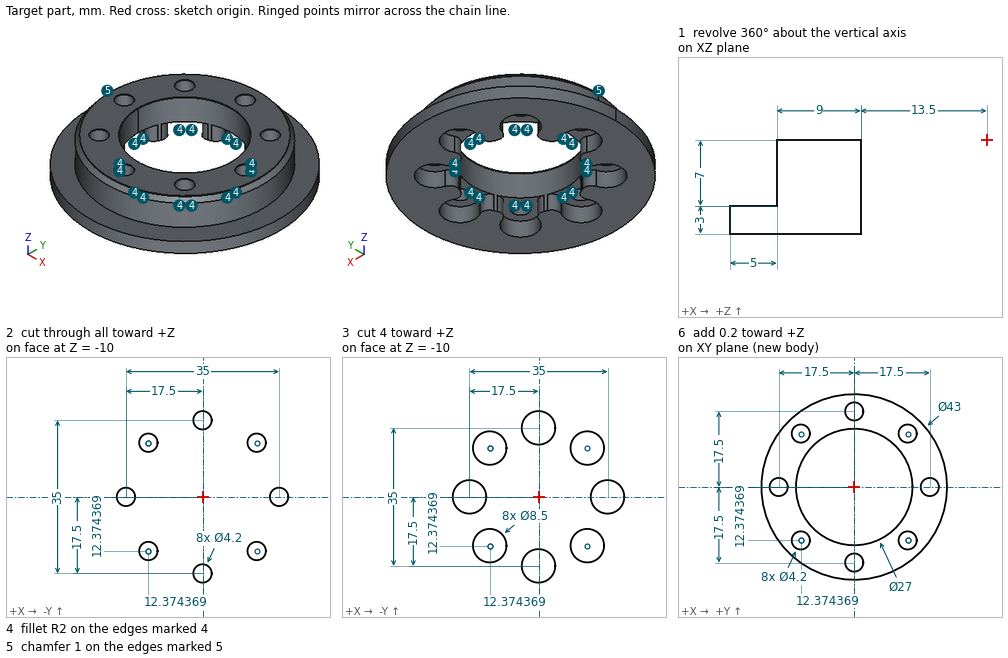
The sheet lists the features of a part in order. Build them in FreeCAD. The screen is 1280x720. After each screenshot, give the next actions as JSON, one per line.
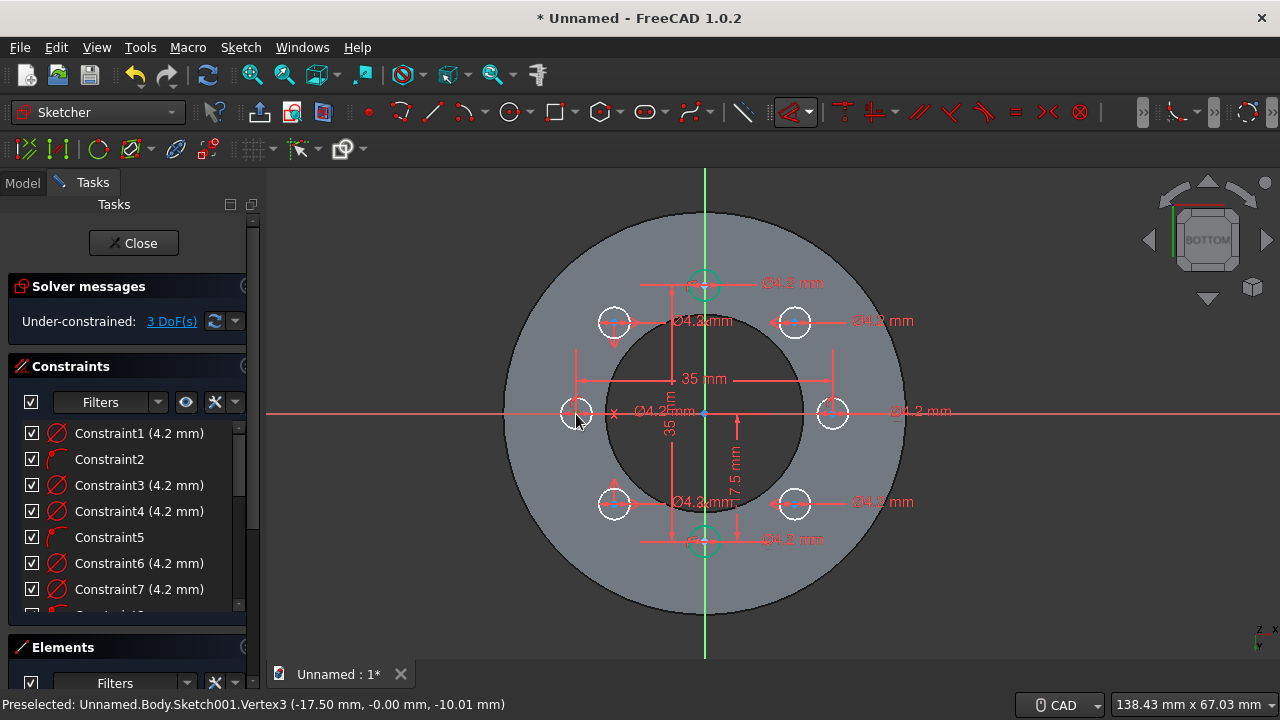
{"action": "left_click", "coordinate": [812, 112]}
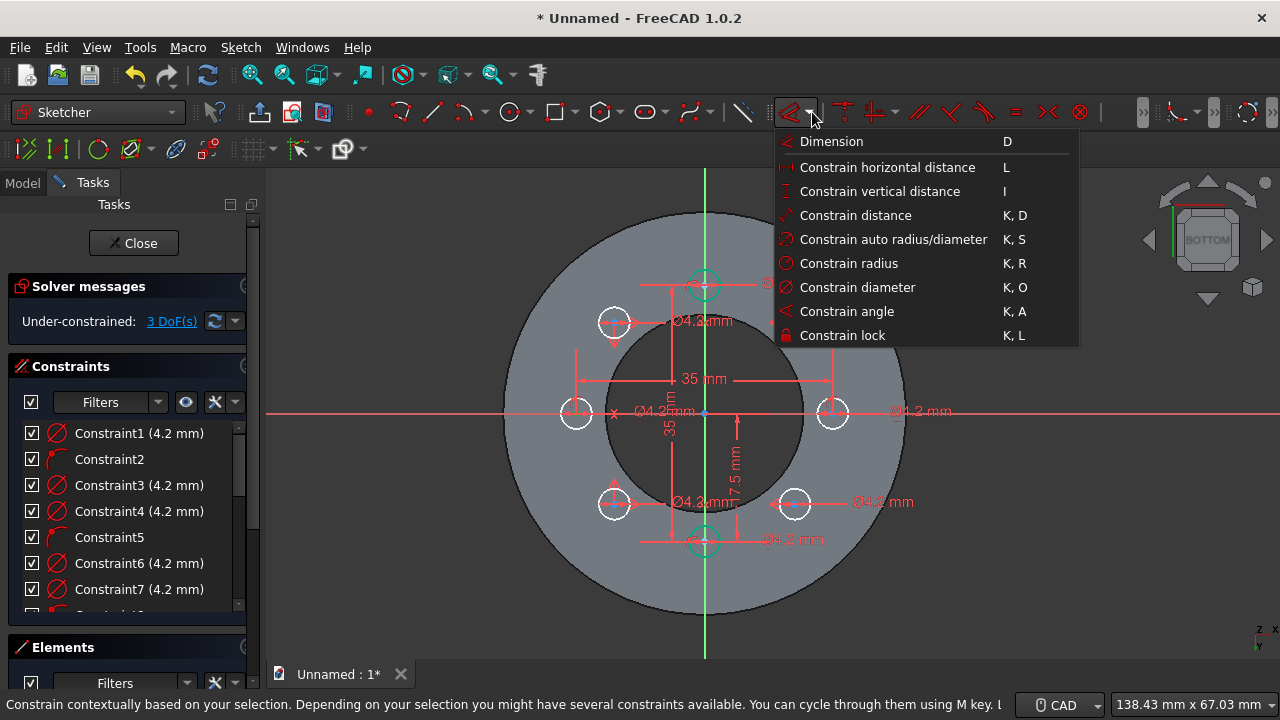
{"action": "left_click", "coordinate": [927, 167]}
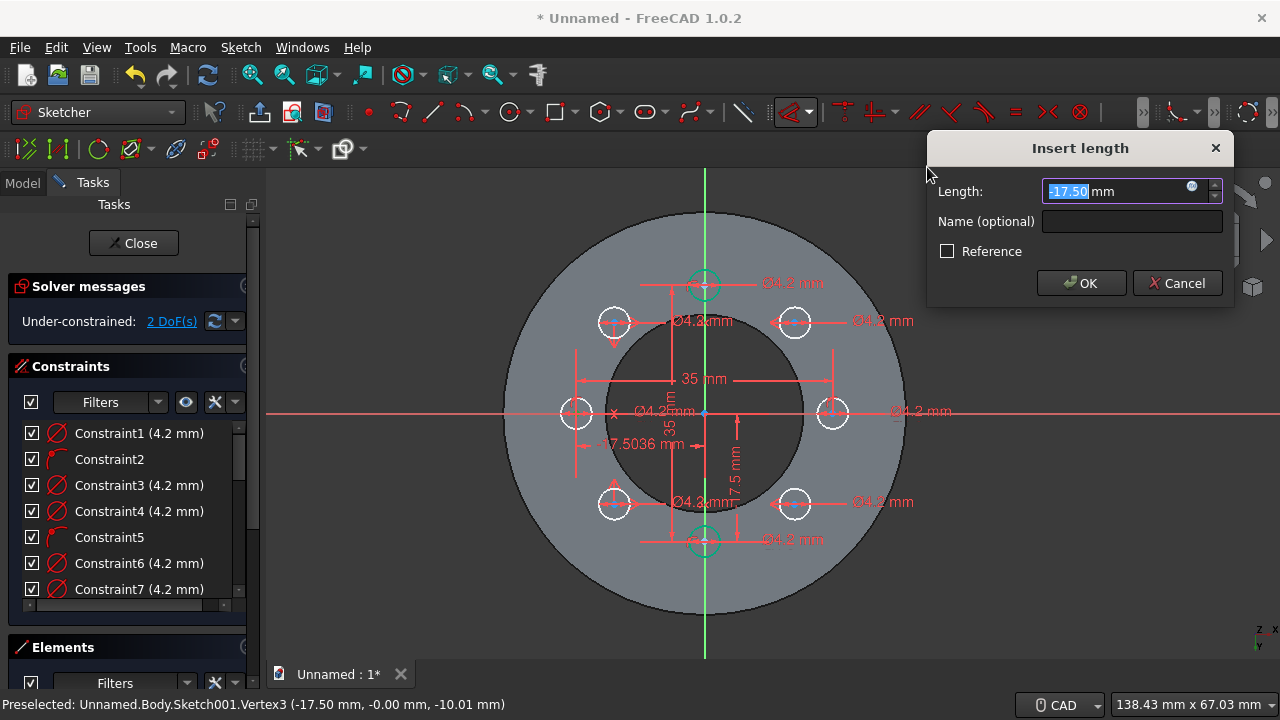
{"action": "type", "text": "-17.5"}
{"action": "key", "text": "Return"}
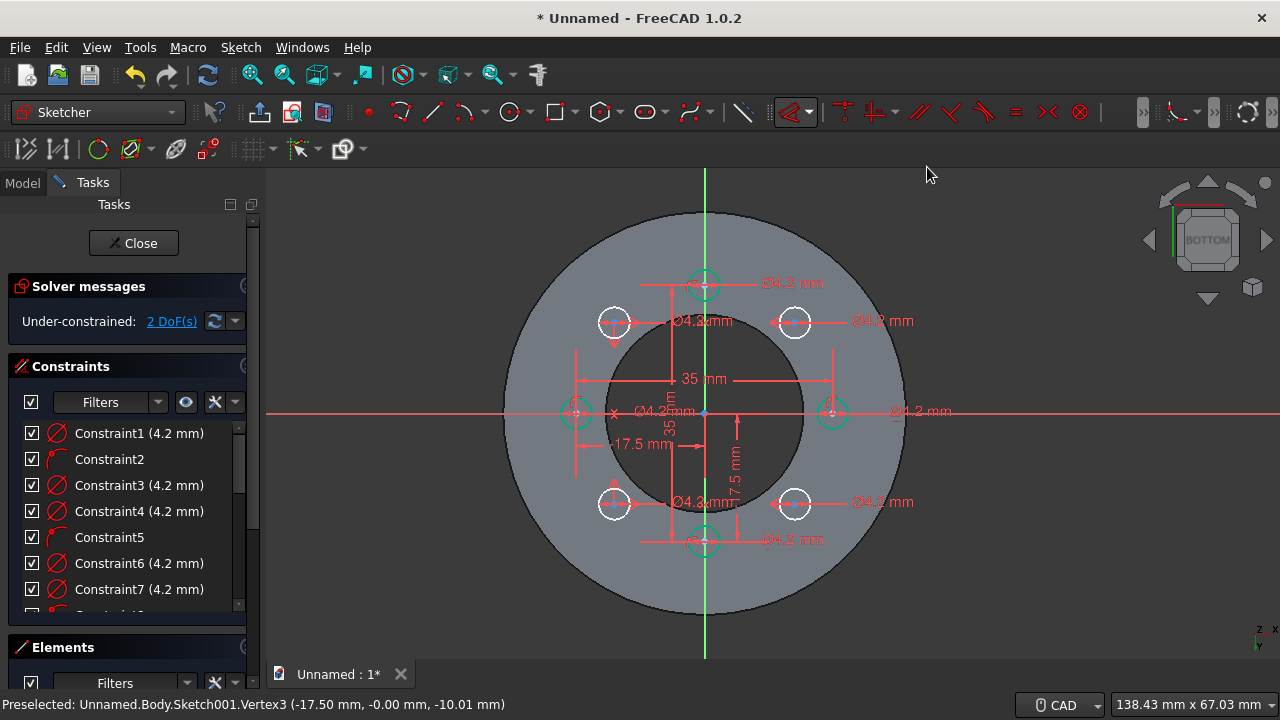
{"action": "left_click", "coordinate": [614, 504]}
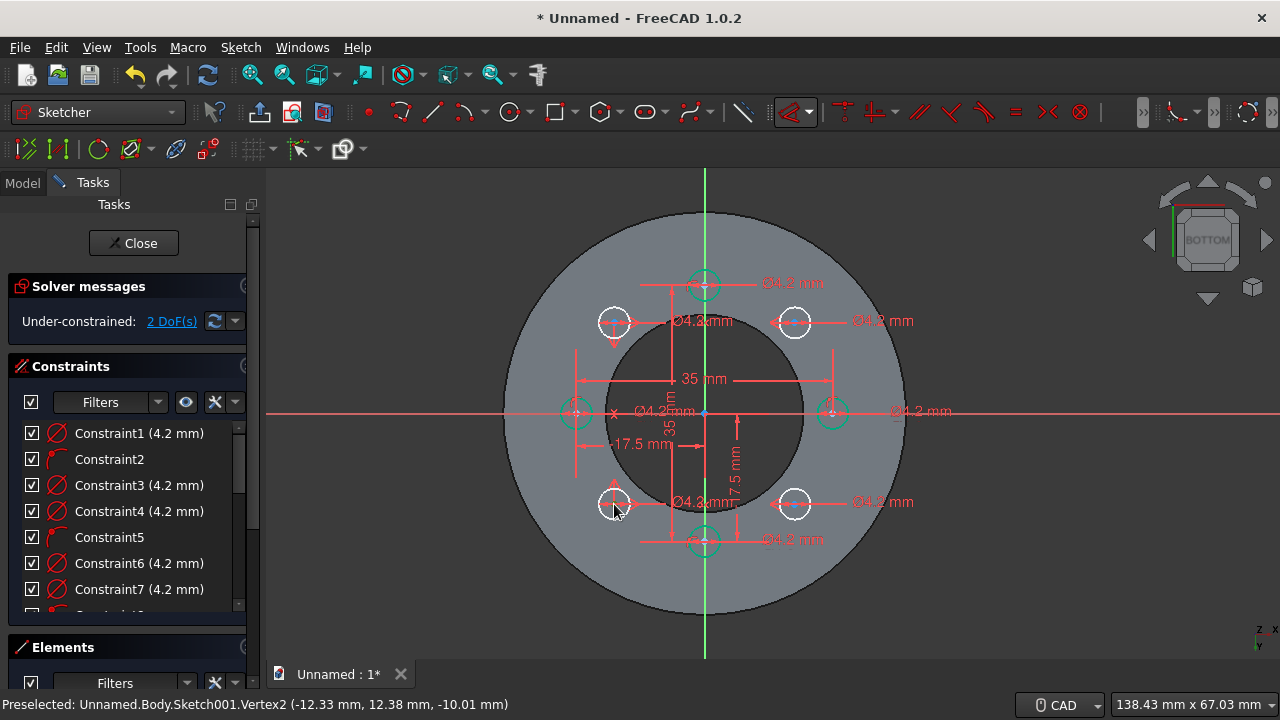
{"action": "key", "text": "l"}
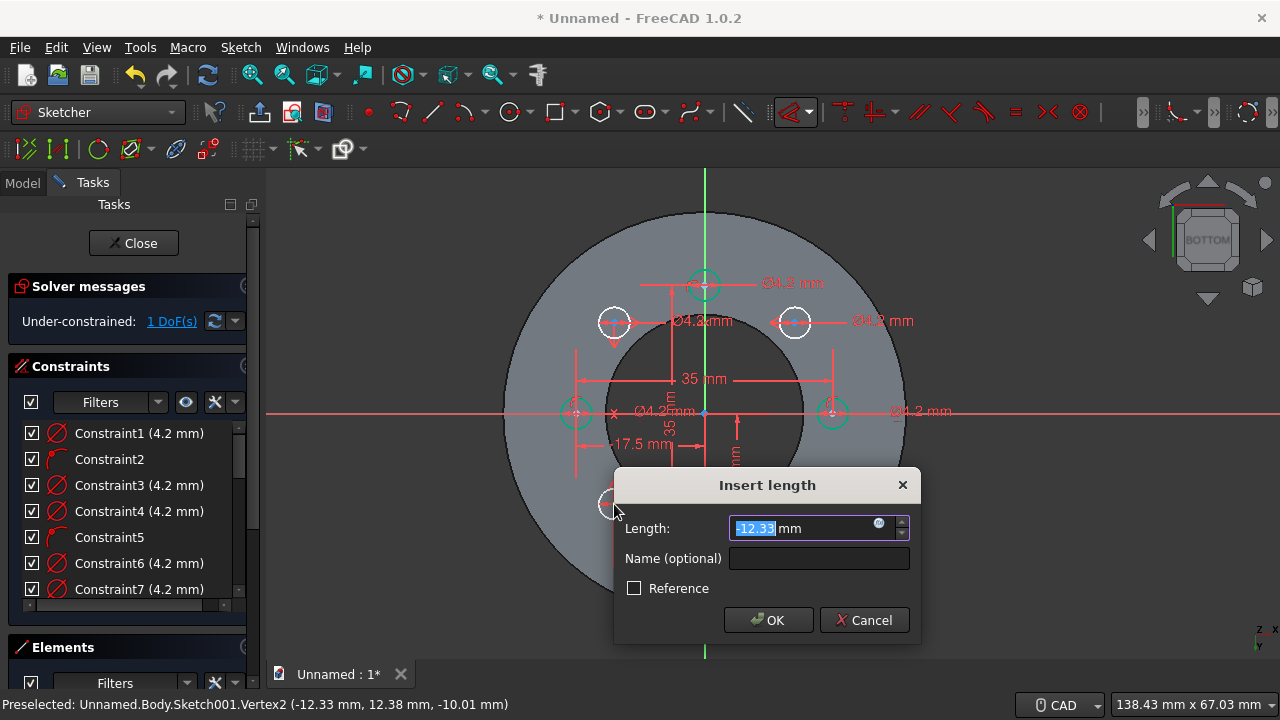
{"action": "type", "text": "-12.374369"}
{"action": "key", "text": "Return"}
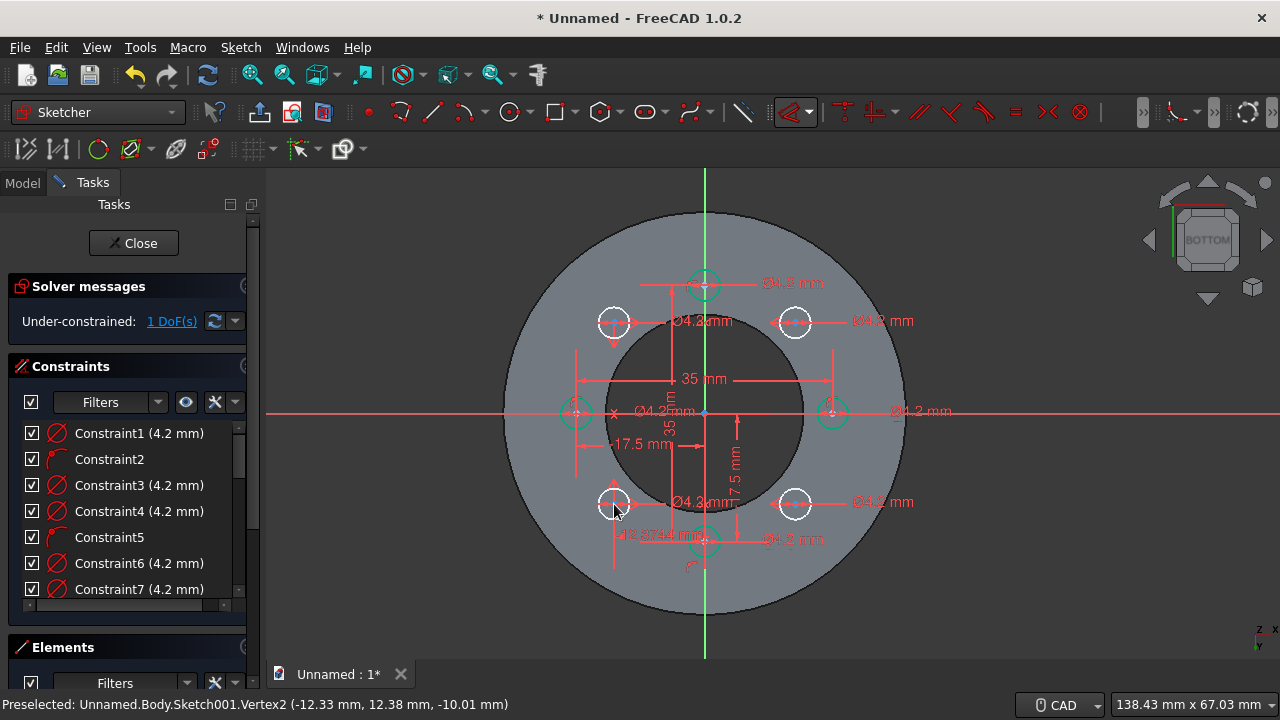
{"action": "left_click", "coordinate": [614, 504]}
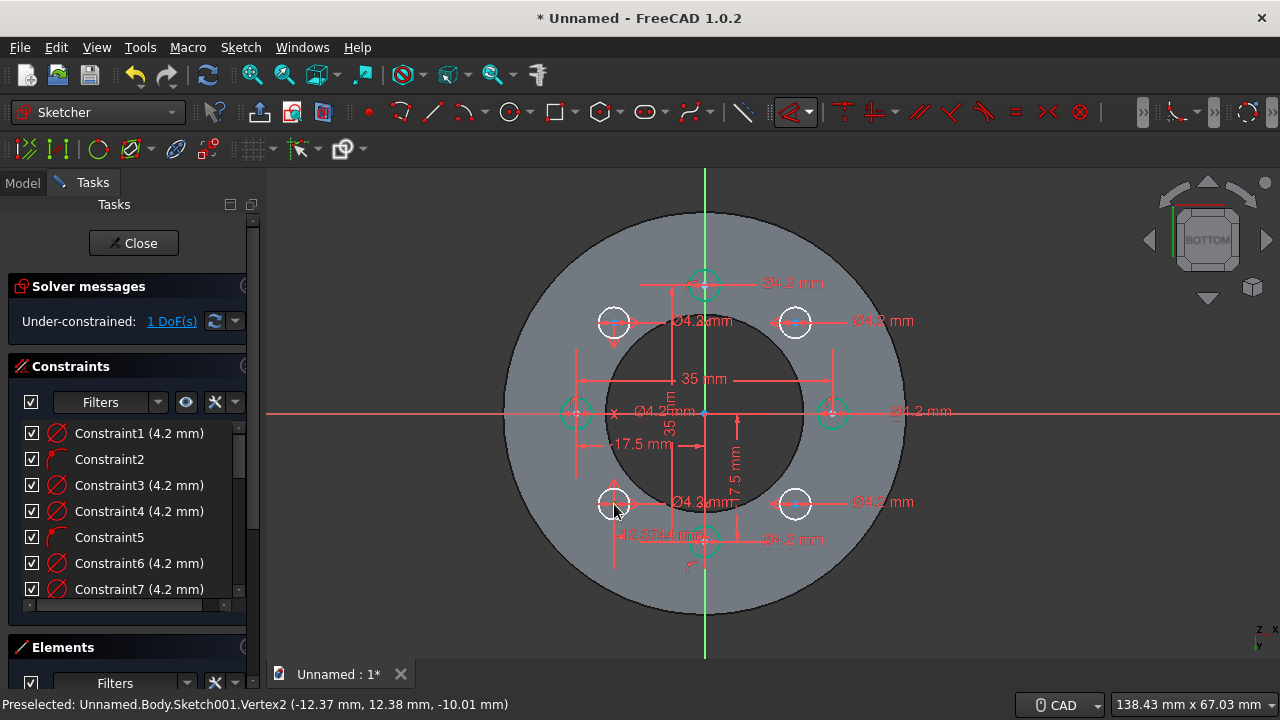
{"action": "key", "text": "i"}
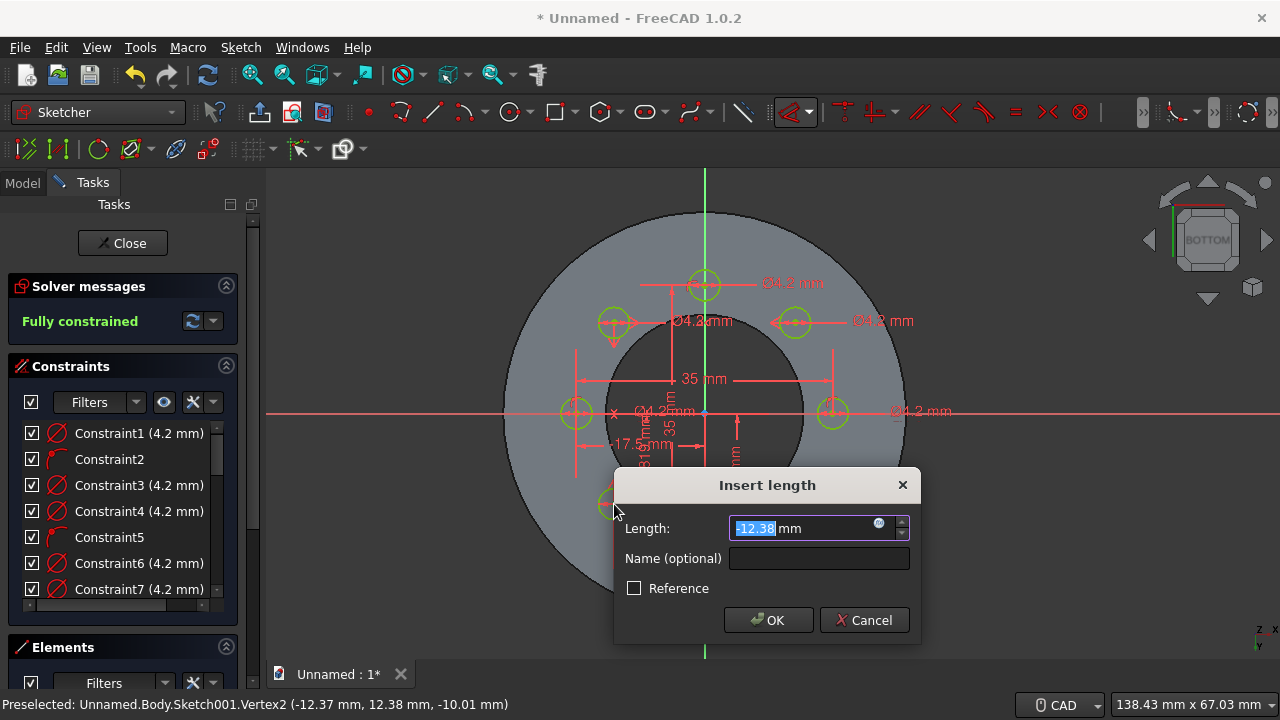
{"action": "type", "text": "-12.374369"}
{"action": "key", "text": "Return"}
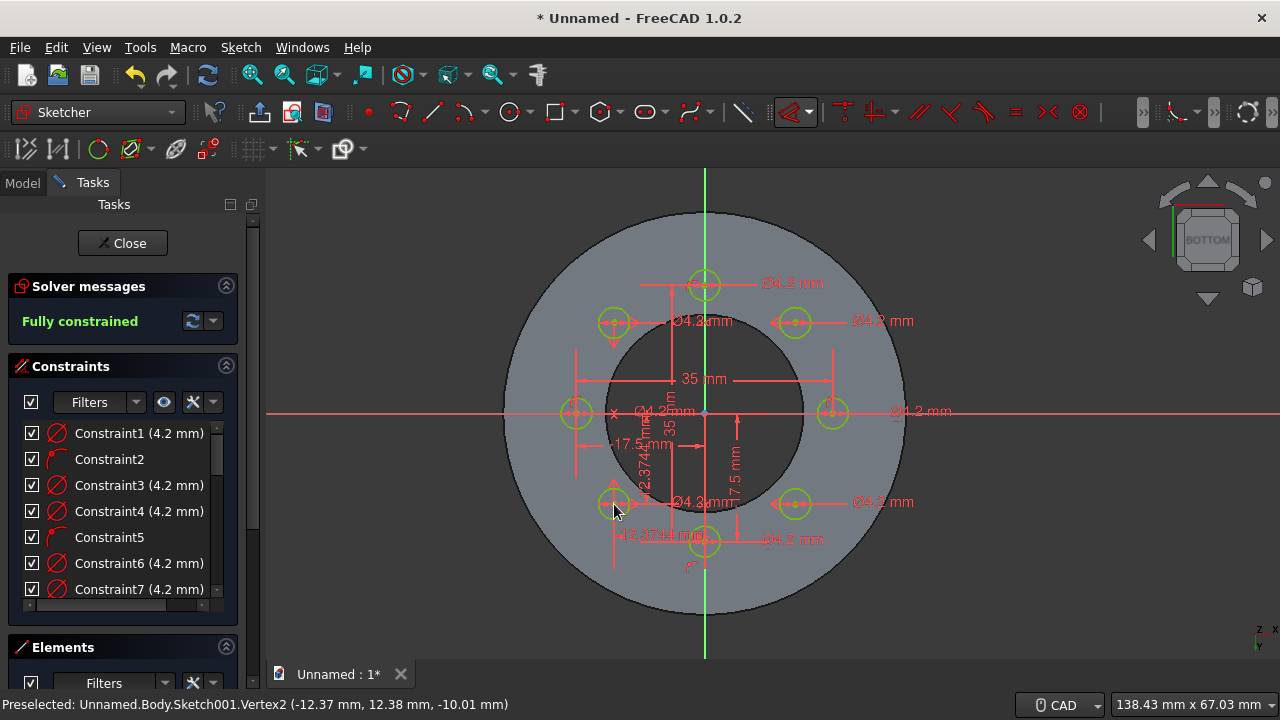
{"action": "left_click", "coordinate": [123, 243]}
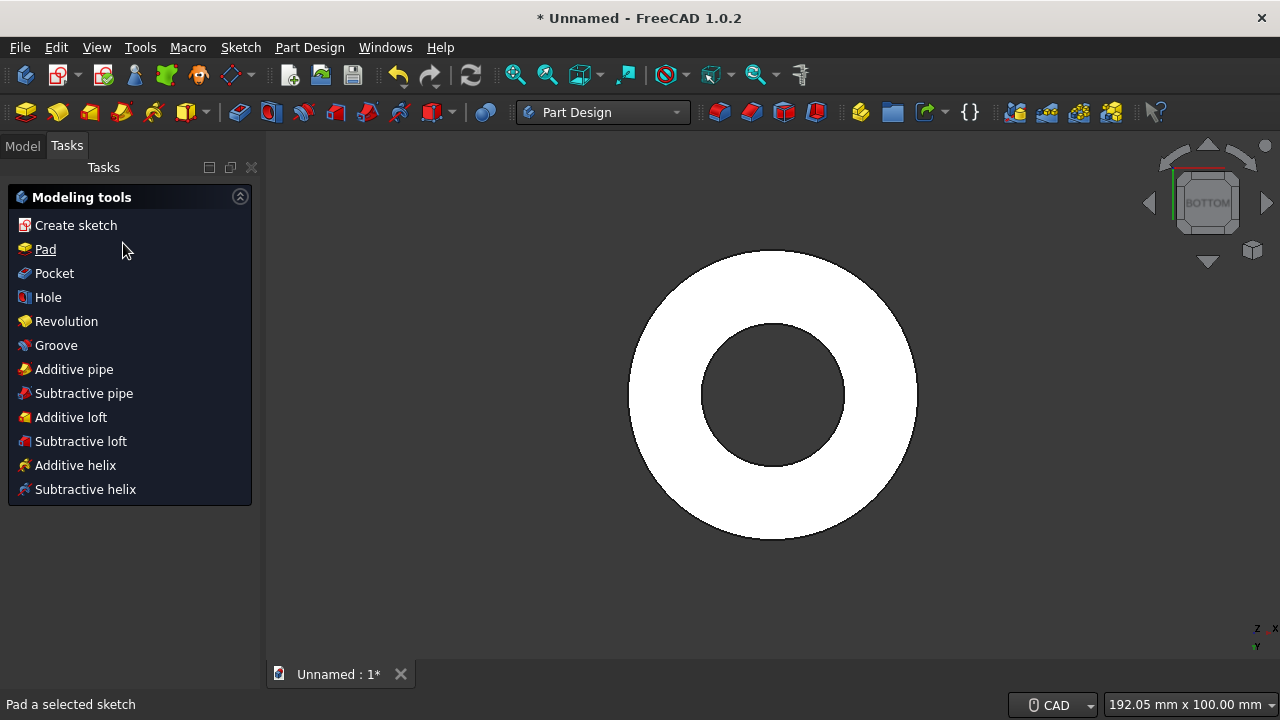
{"action": "left_click", "coordinate": [240, 112]}